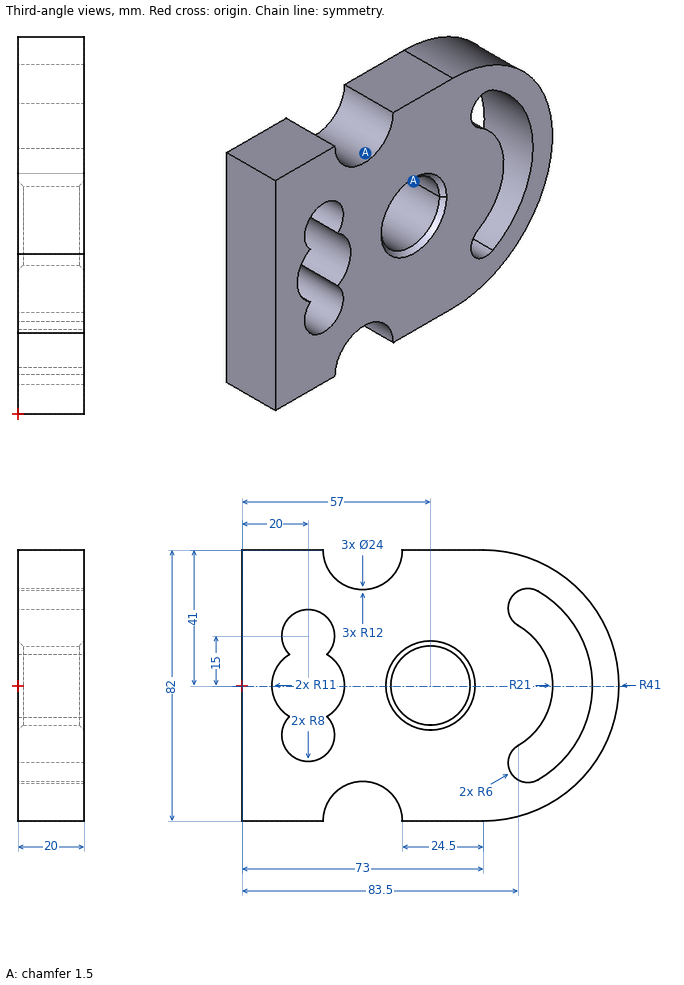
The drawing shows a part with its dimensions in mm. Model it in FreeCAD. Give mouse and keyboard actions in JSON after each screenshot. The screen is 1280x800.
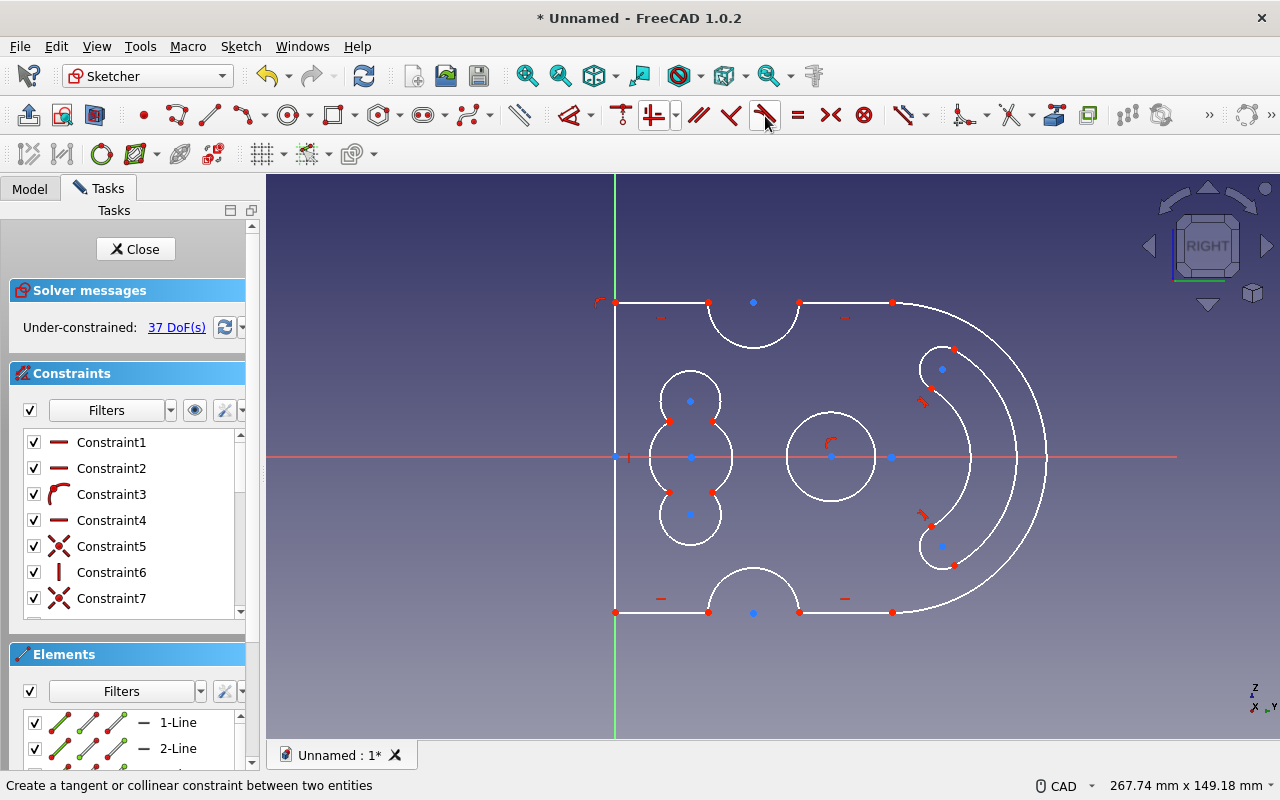
{"action": "left_click", "coordinate": [933, 349]}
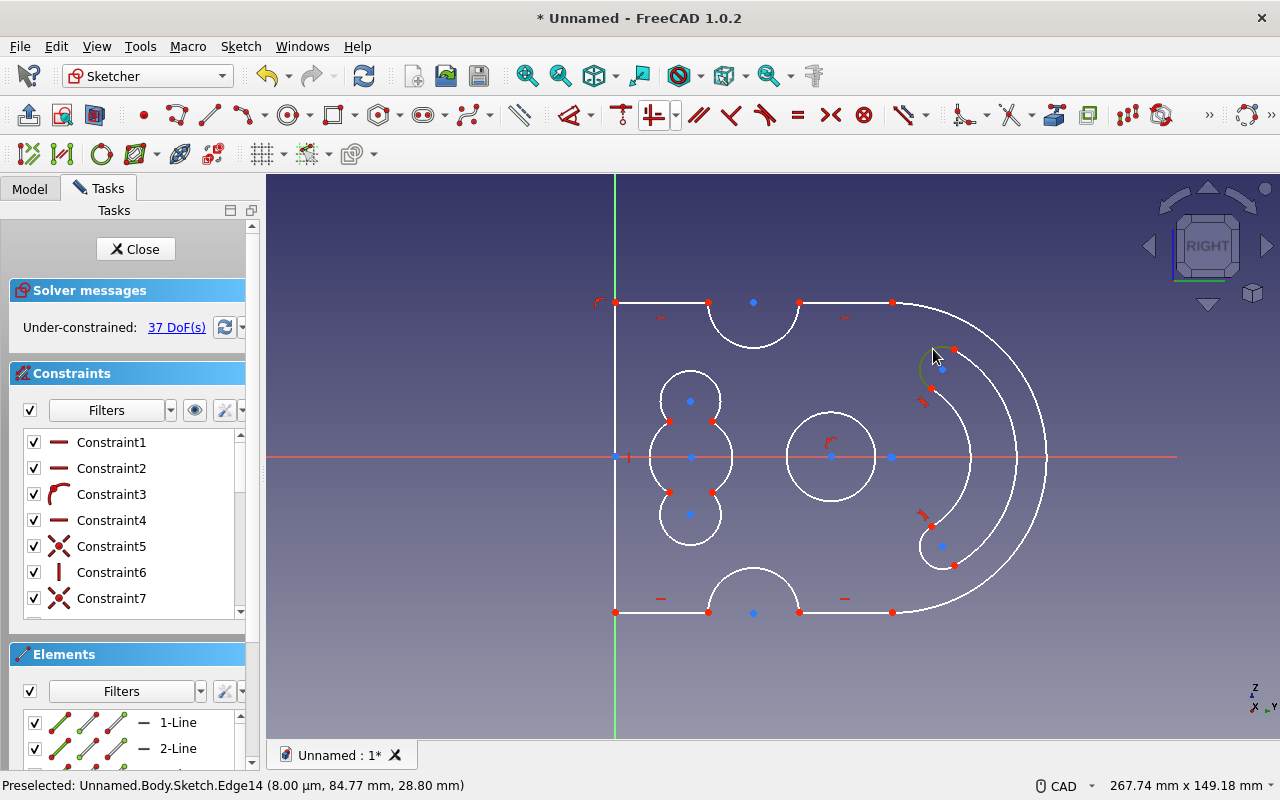
{"action": "left_click", "coordinate": [1006, 509]}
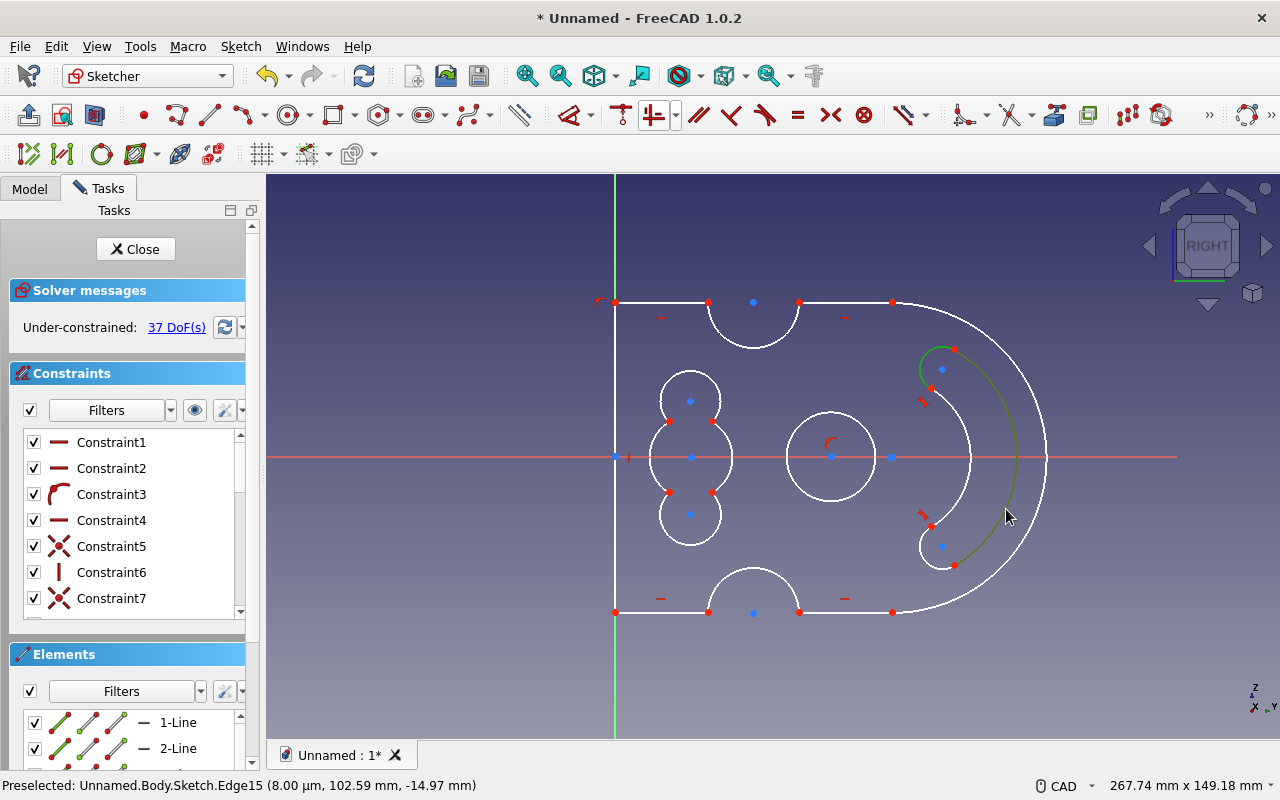
{"action": "key", "text": "t"}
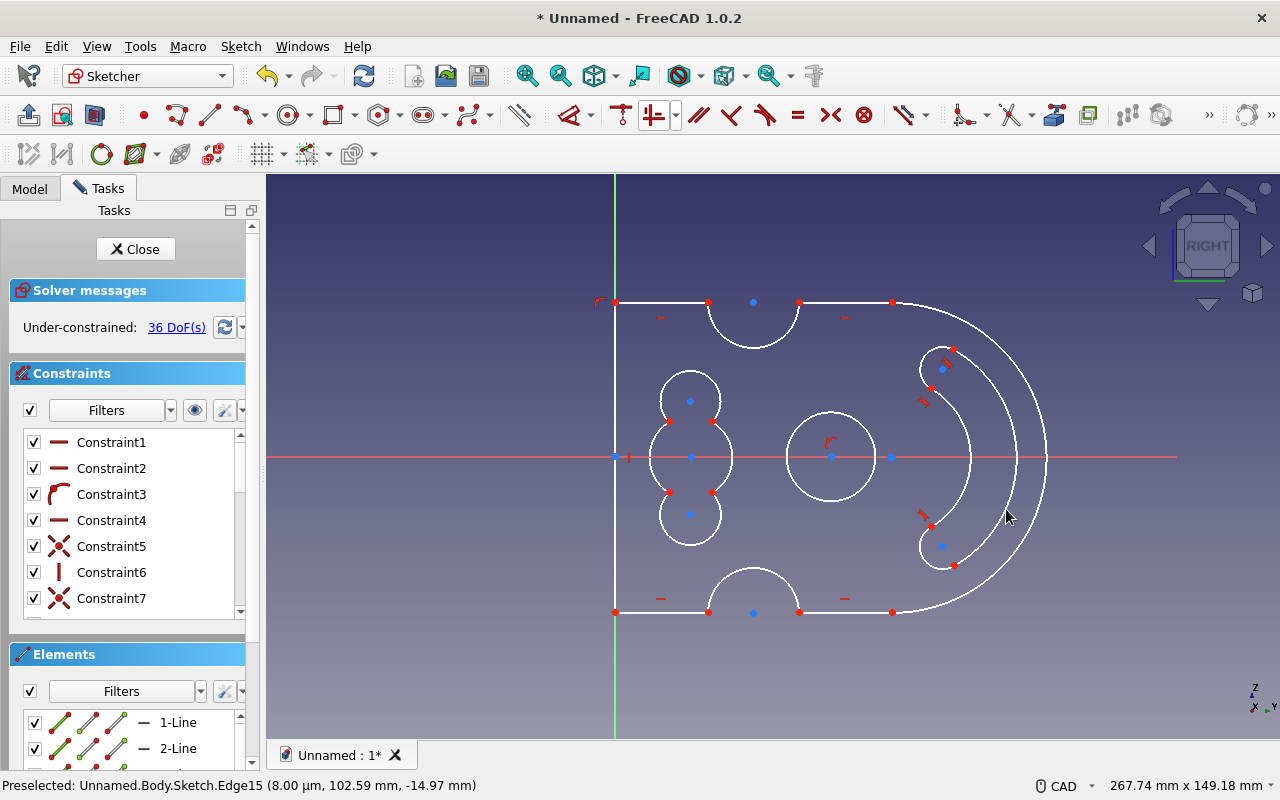
{"action": "left_click", "coordinate": [1006, 509]}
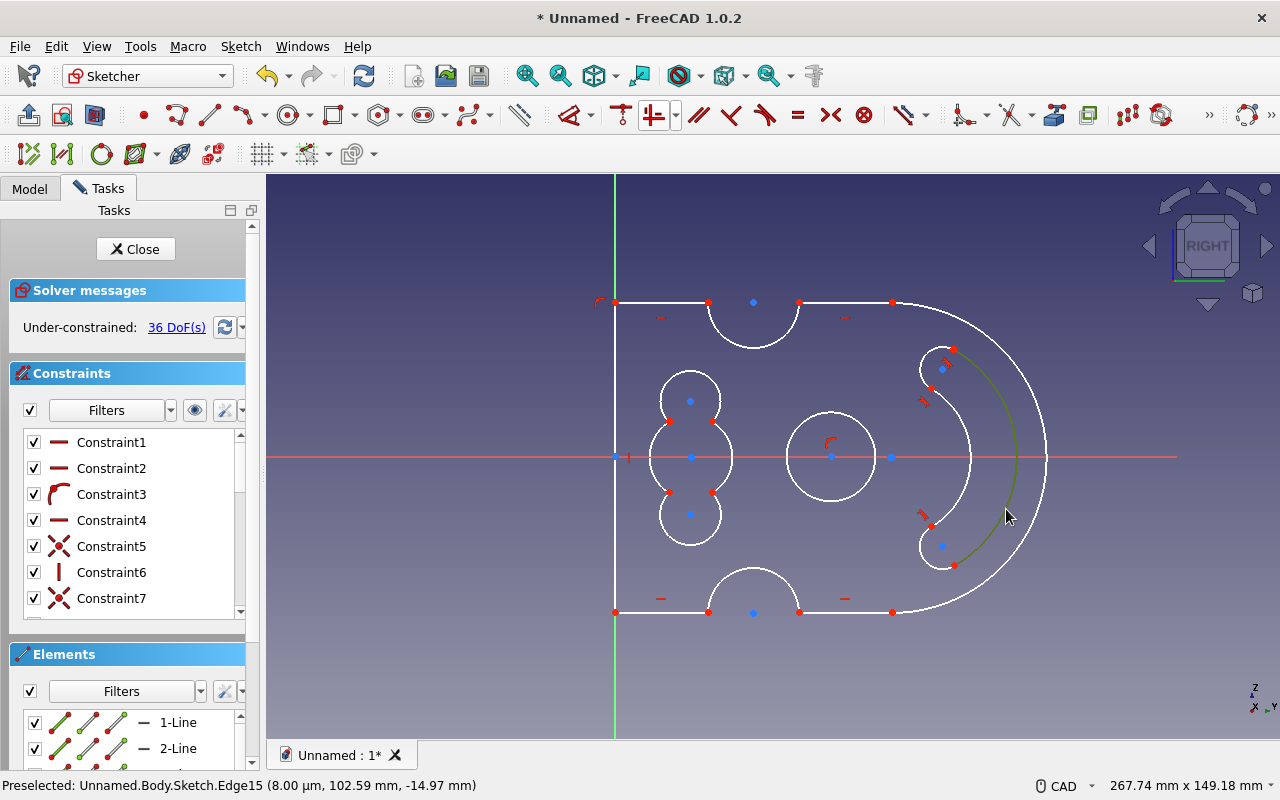
{"action": "left_click", "coordinate": [920, 544]}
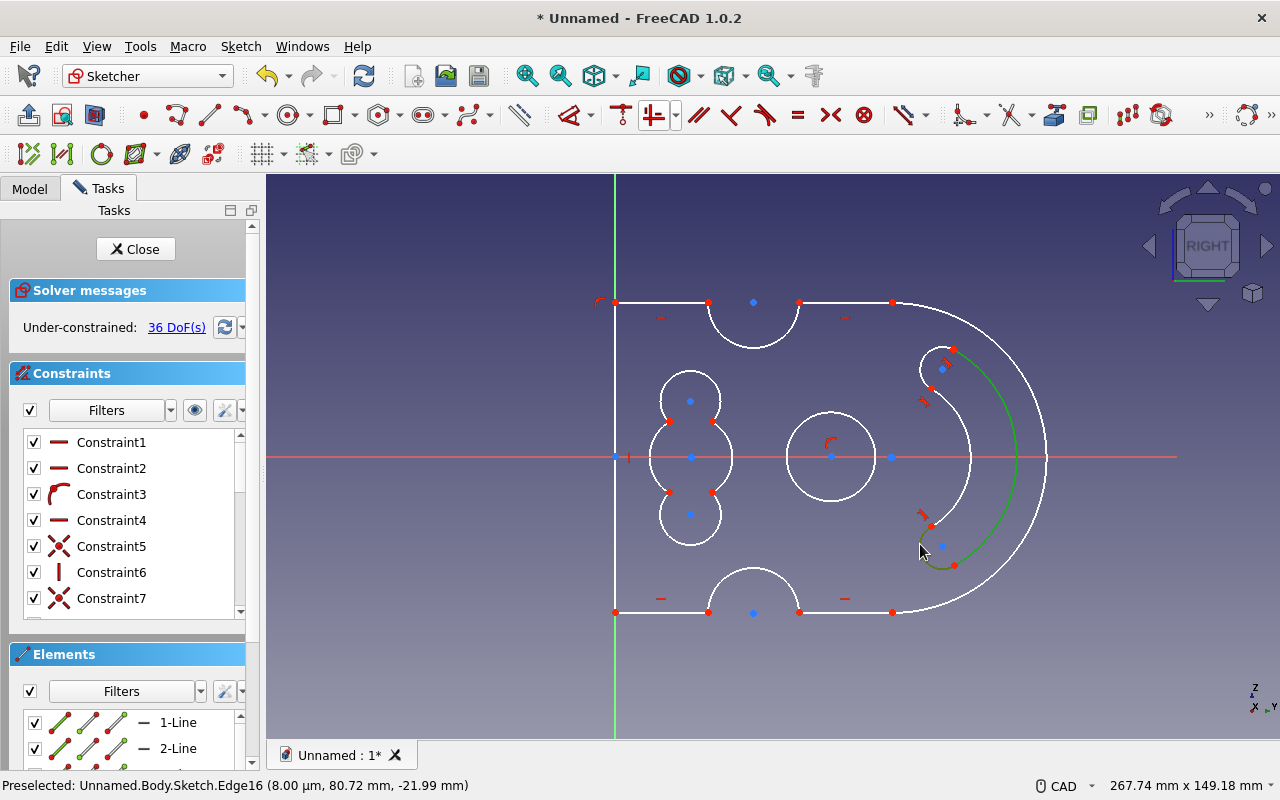
{"action": "key", "text": "t"}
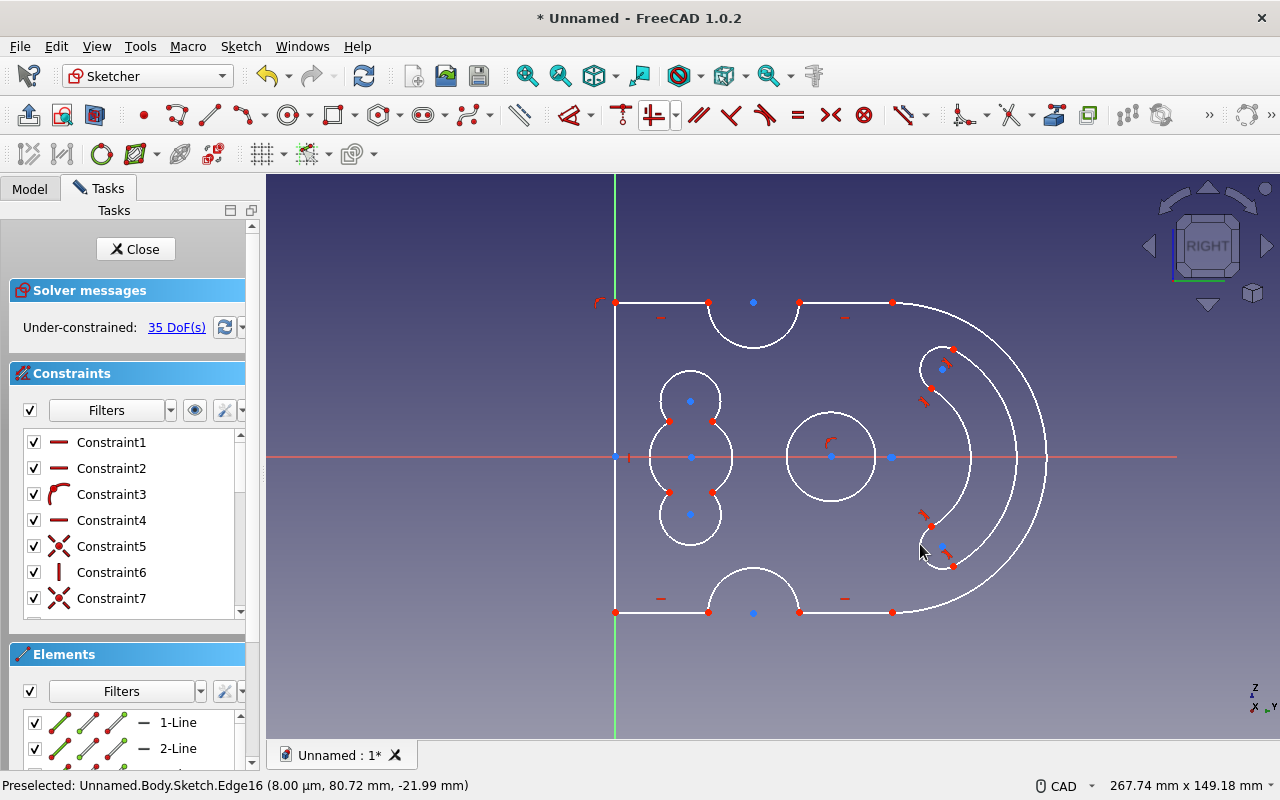
{"action": "left_click", "coordinate": [653, 441]}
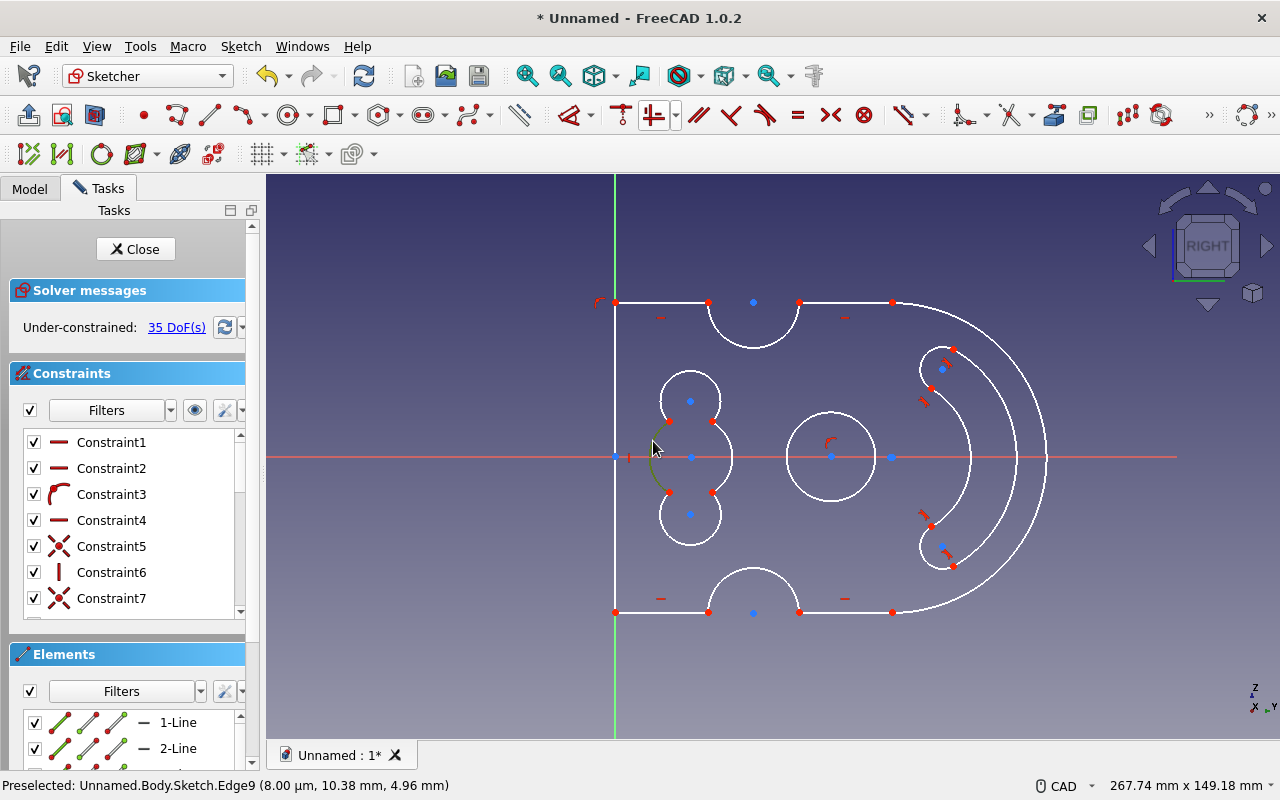
{"action": "left_click", "coordinate": [729, 474]}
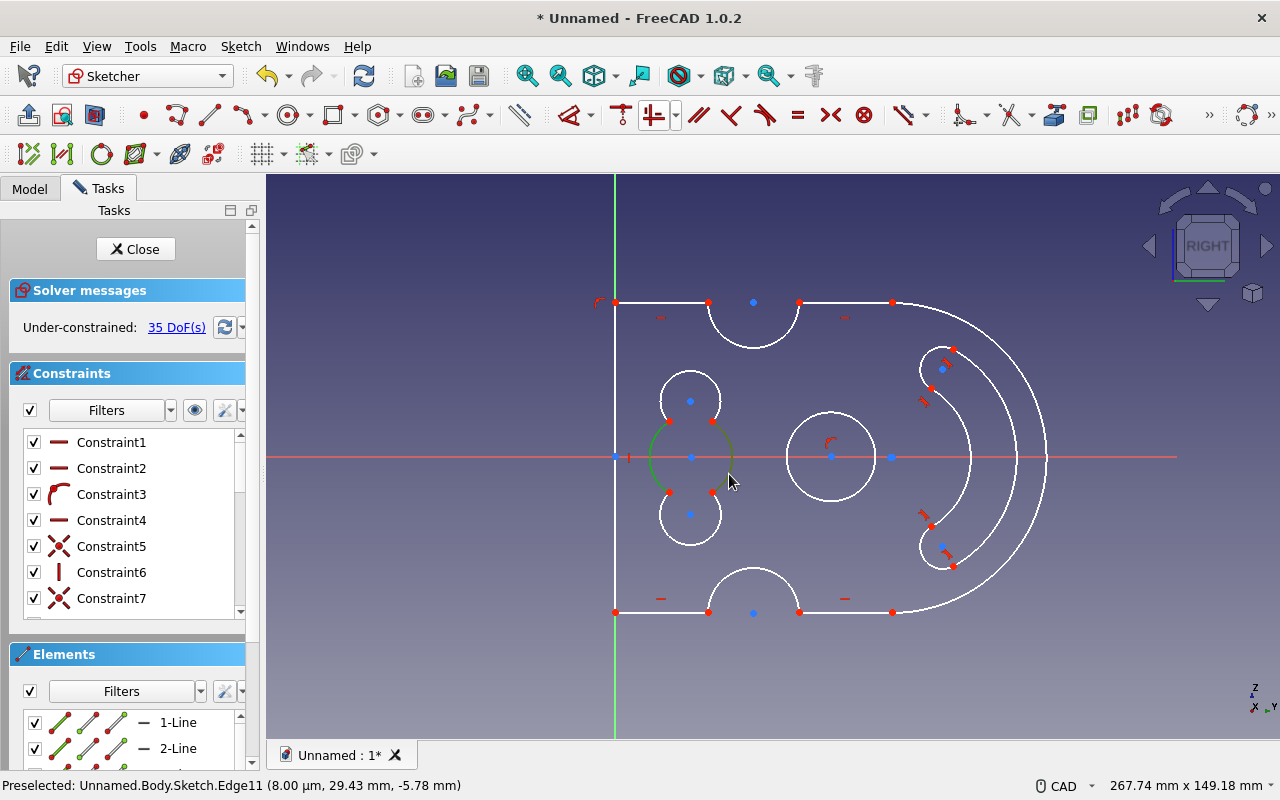
{"action": "key", "text": "c"}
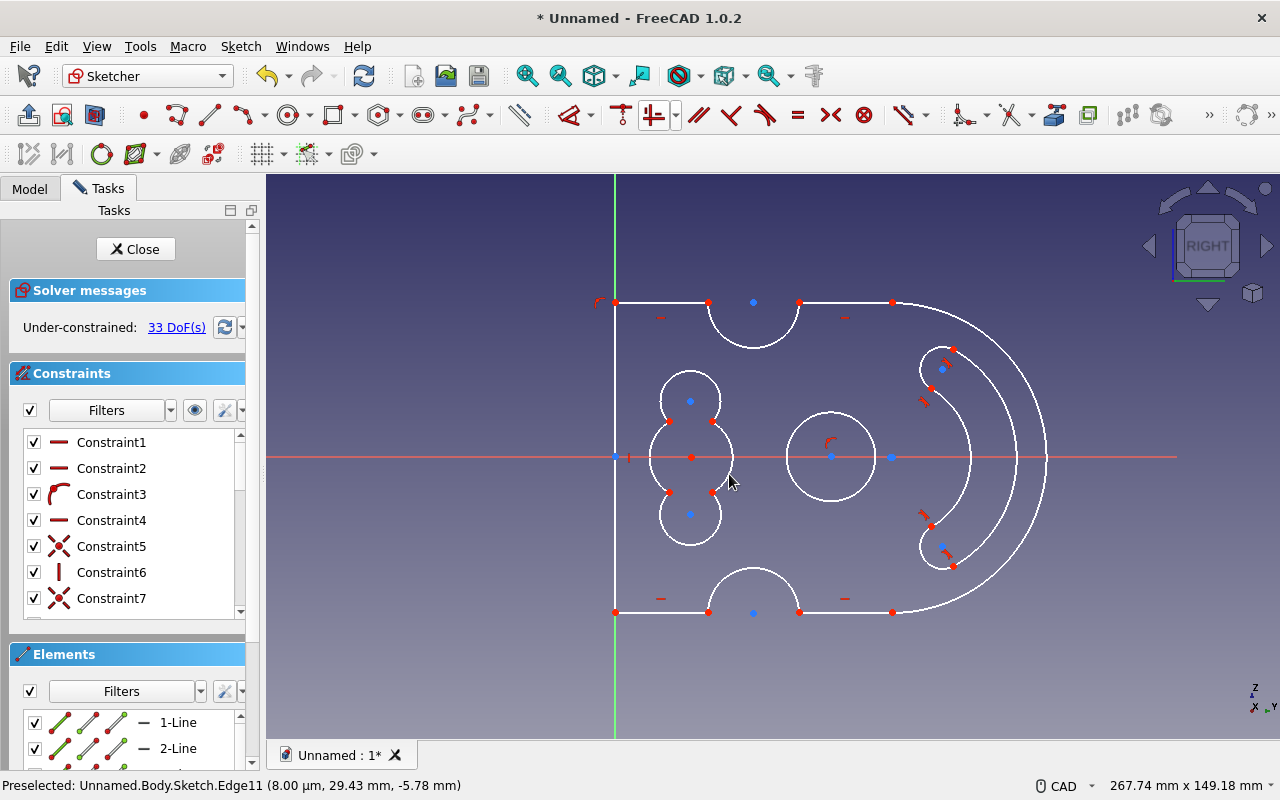
{"action": "left_click", "coordinate": [1017, 549]}